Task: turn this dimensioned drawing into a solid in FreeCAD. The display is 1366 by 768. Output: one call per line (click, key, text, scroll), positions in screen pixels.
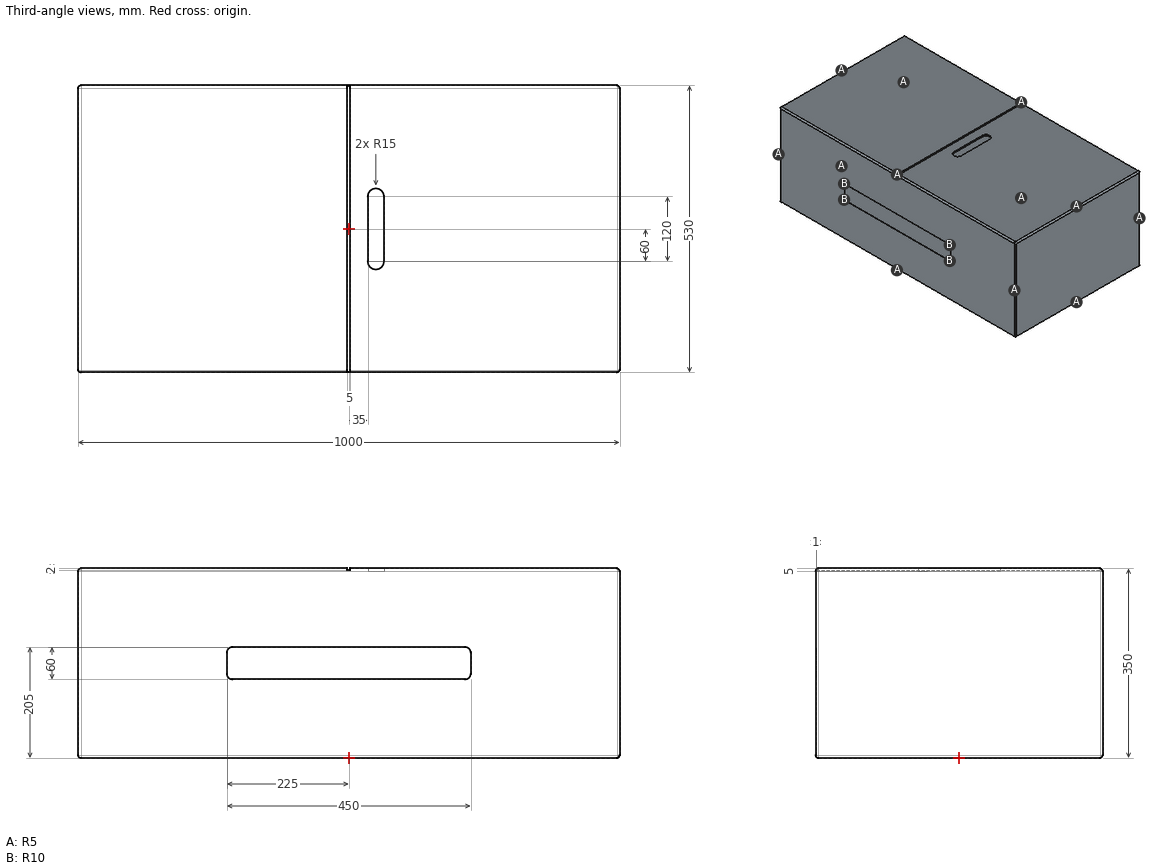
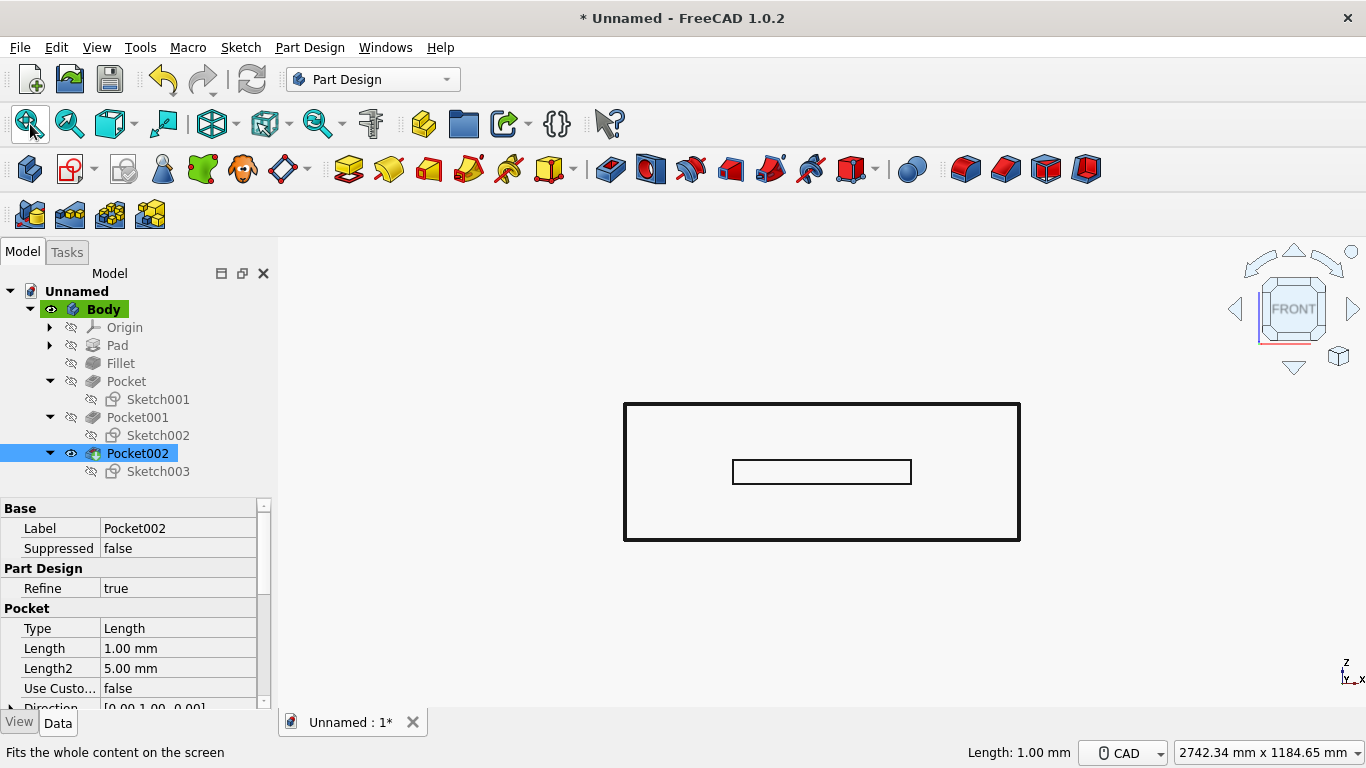
key(3)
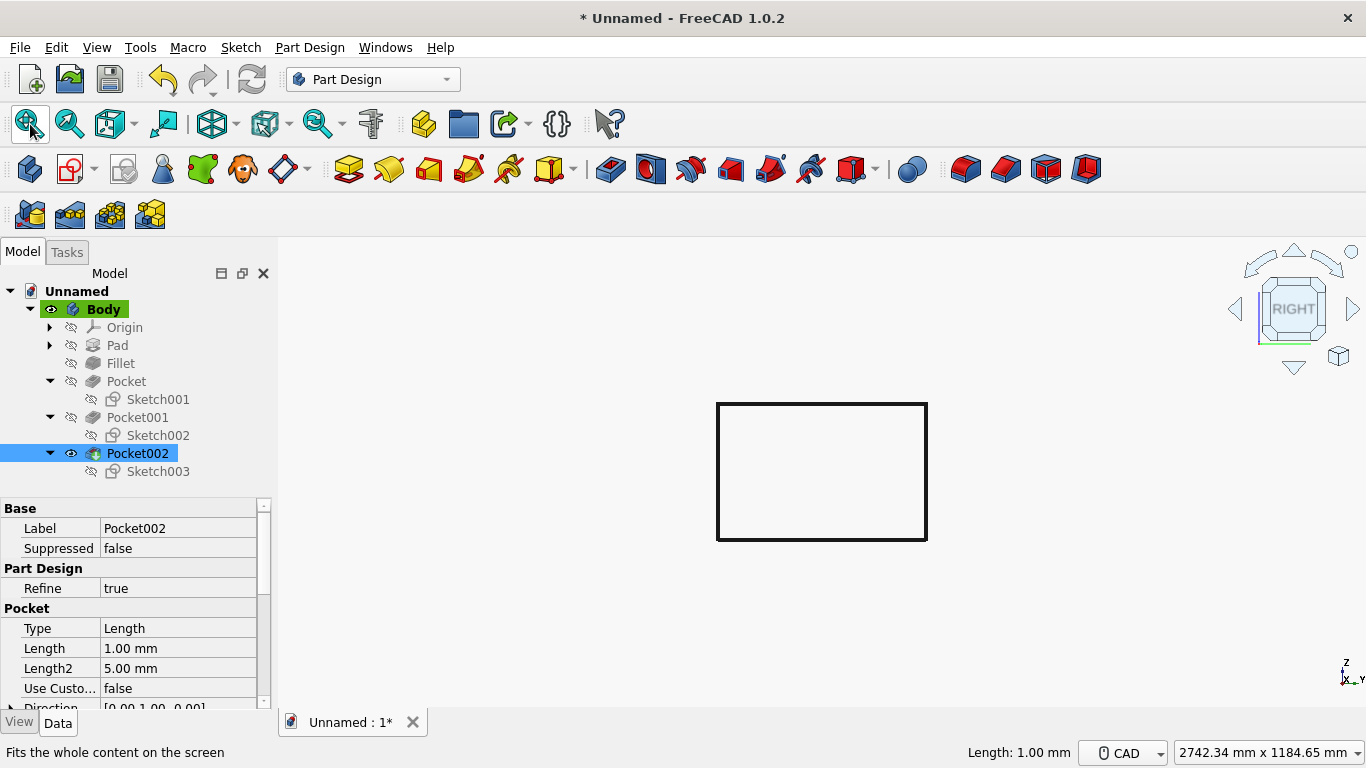
click(30, 124)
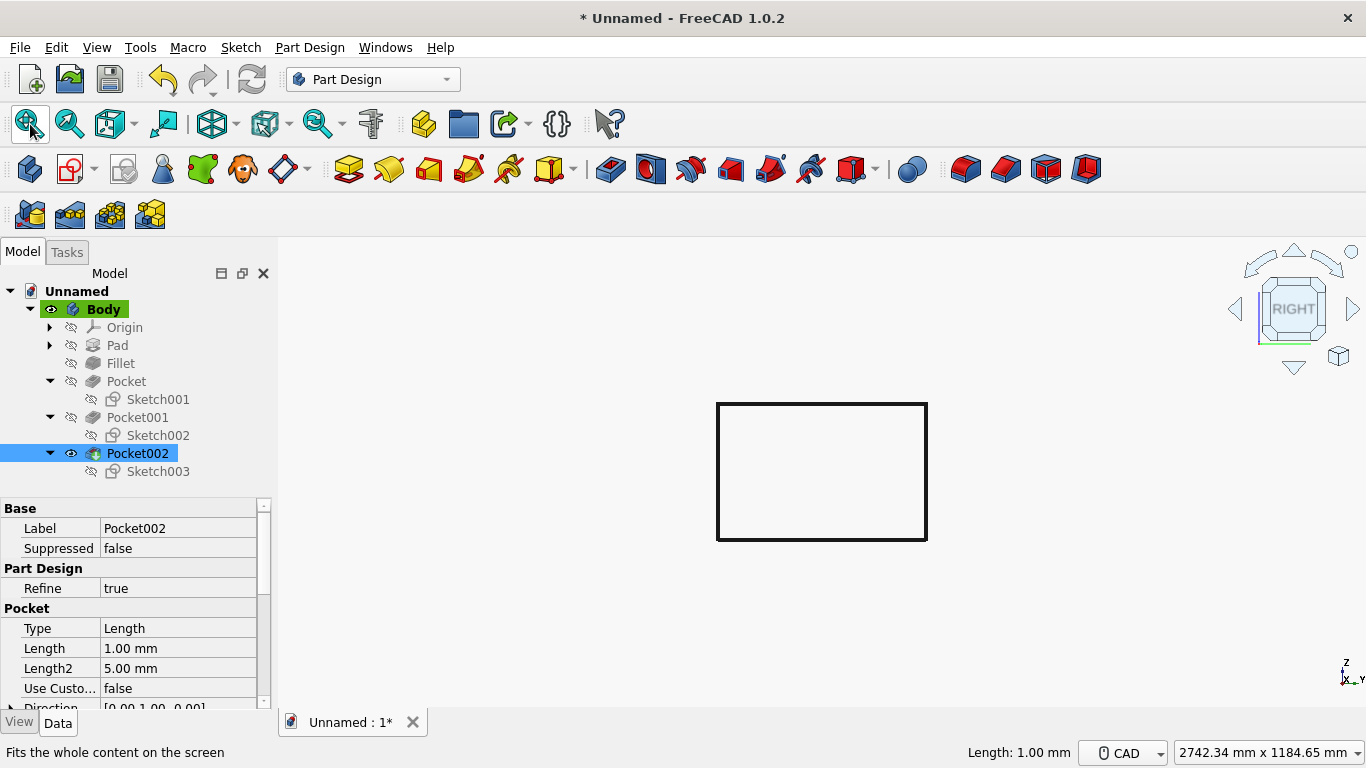
scroll(717, 483, up, 15)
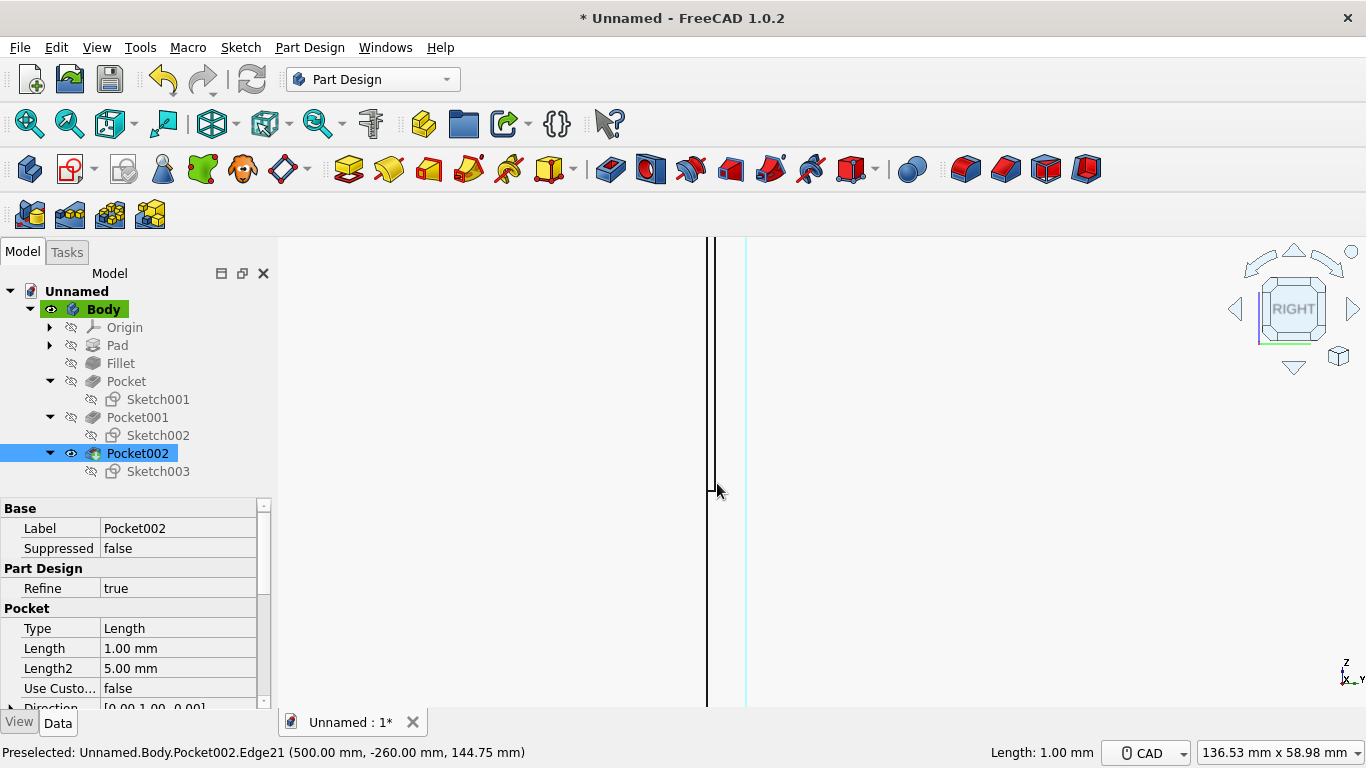
scroll(711, 490, up, 9)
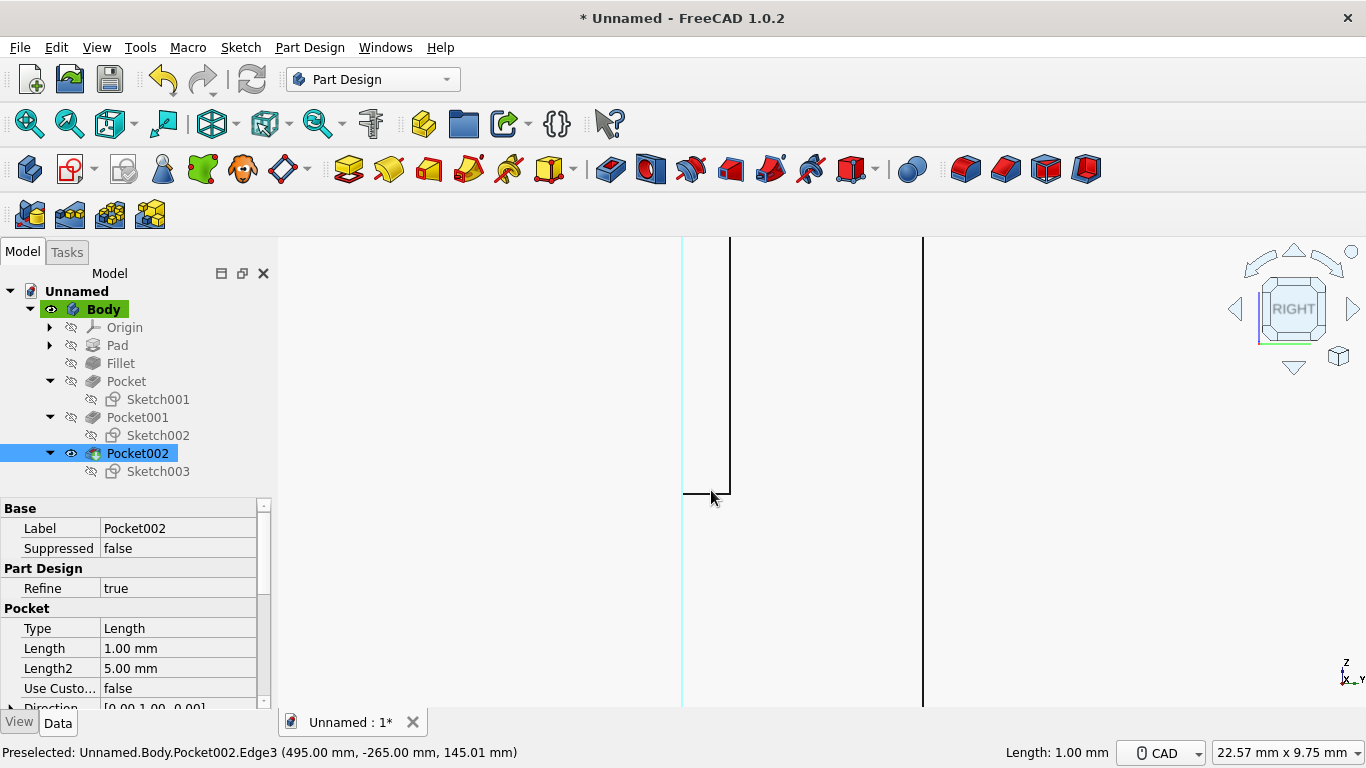
click(706, 493, ctrl)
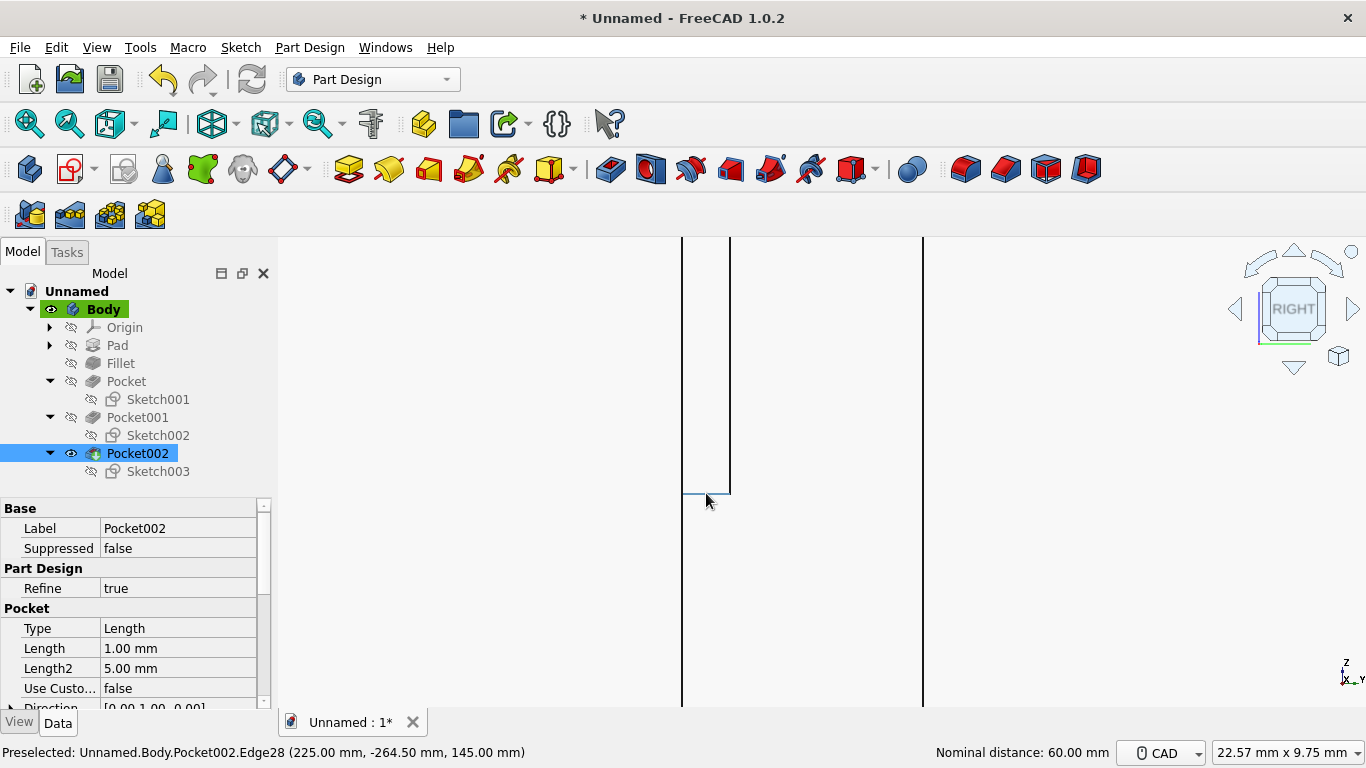
click(30, 124)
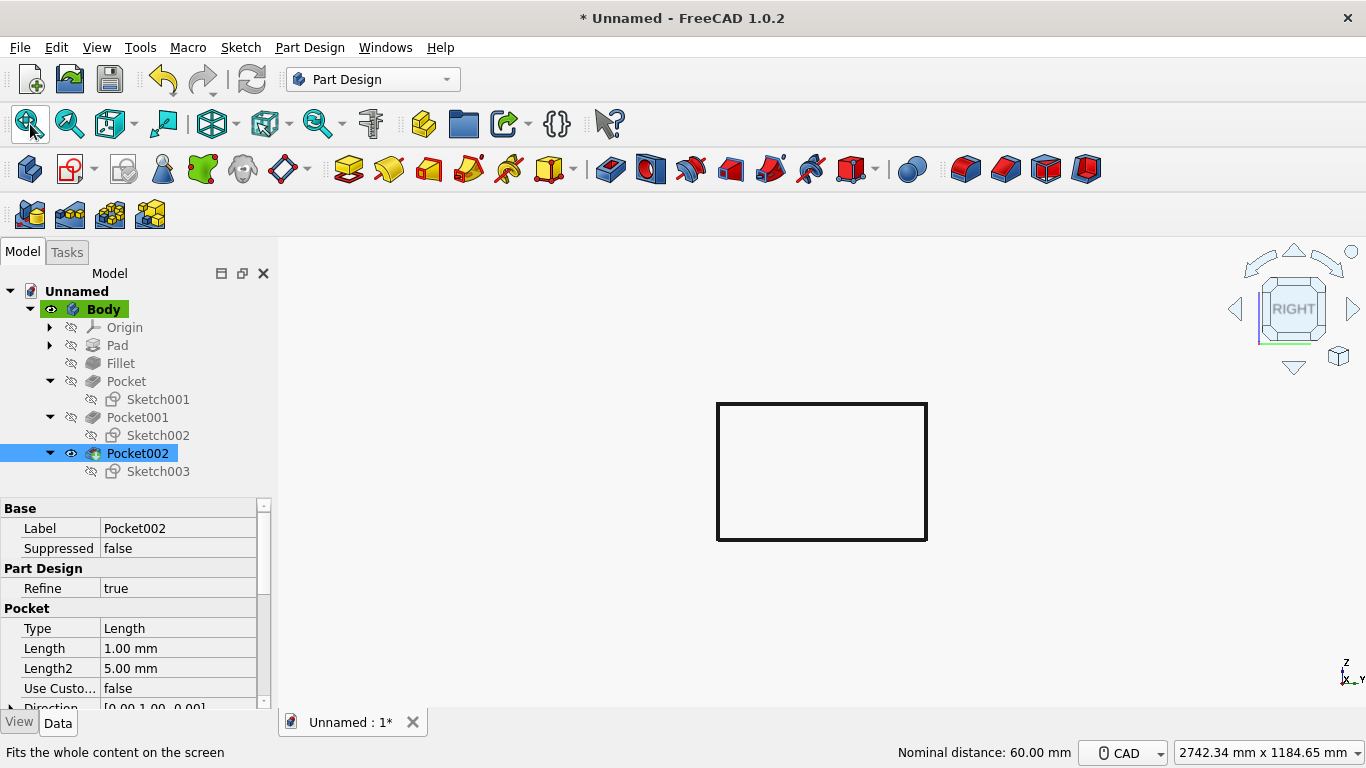
key(5)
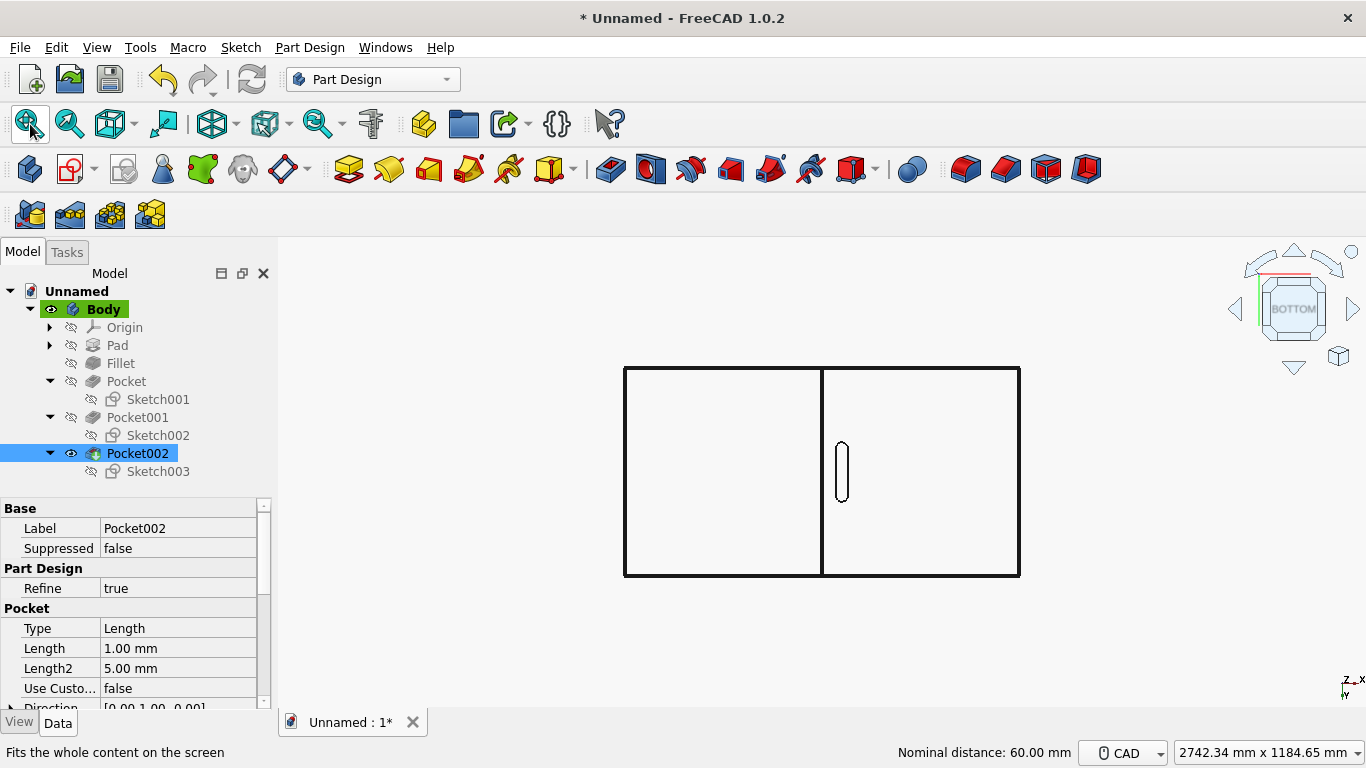
click(30, 124)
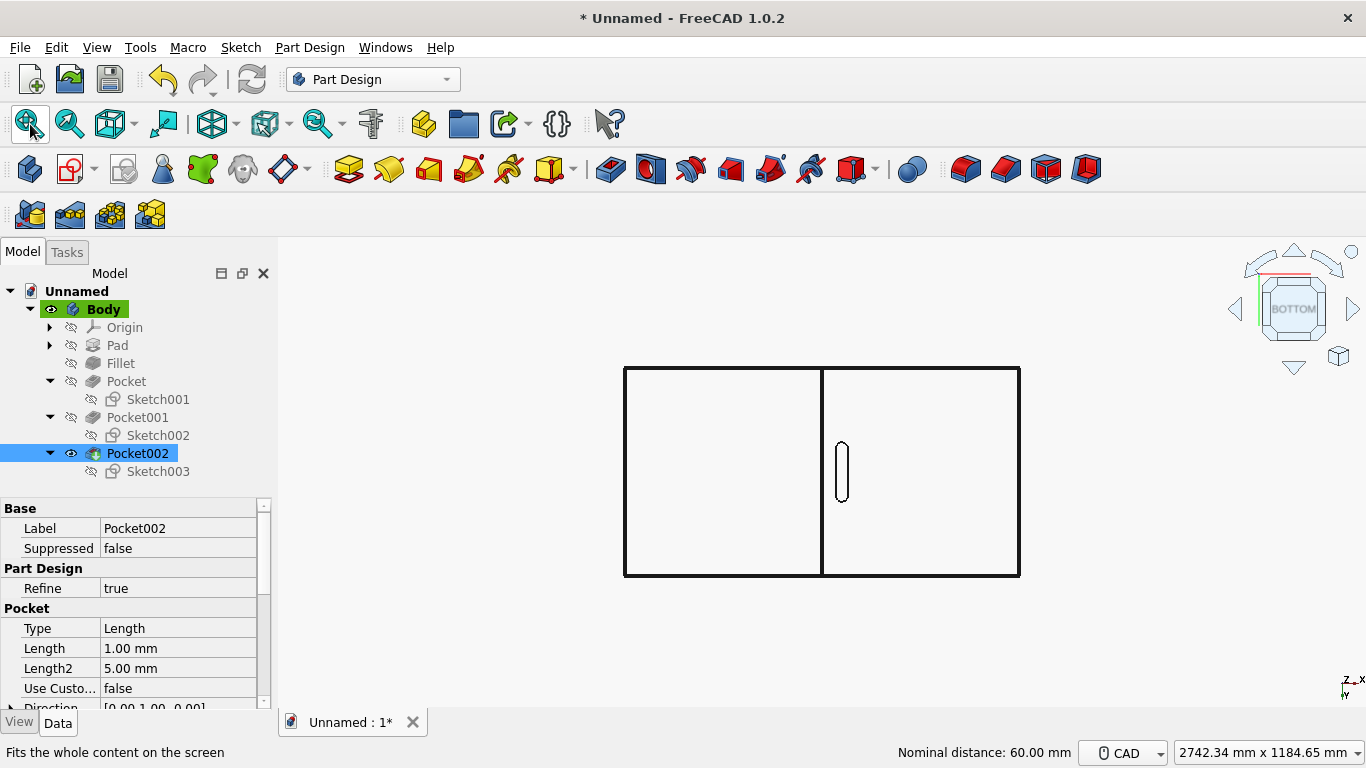
scroll(733, 366, up, 15)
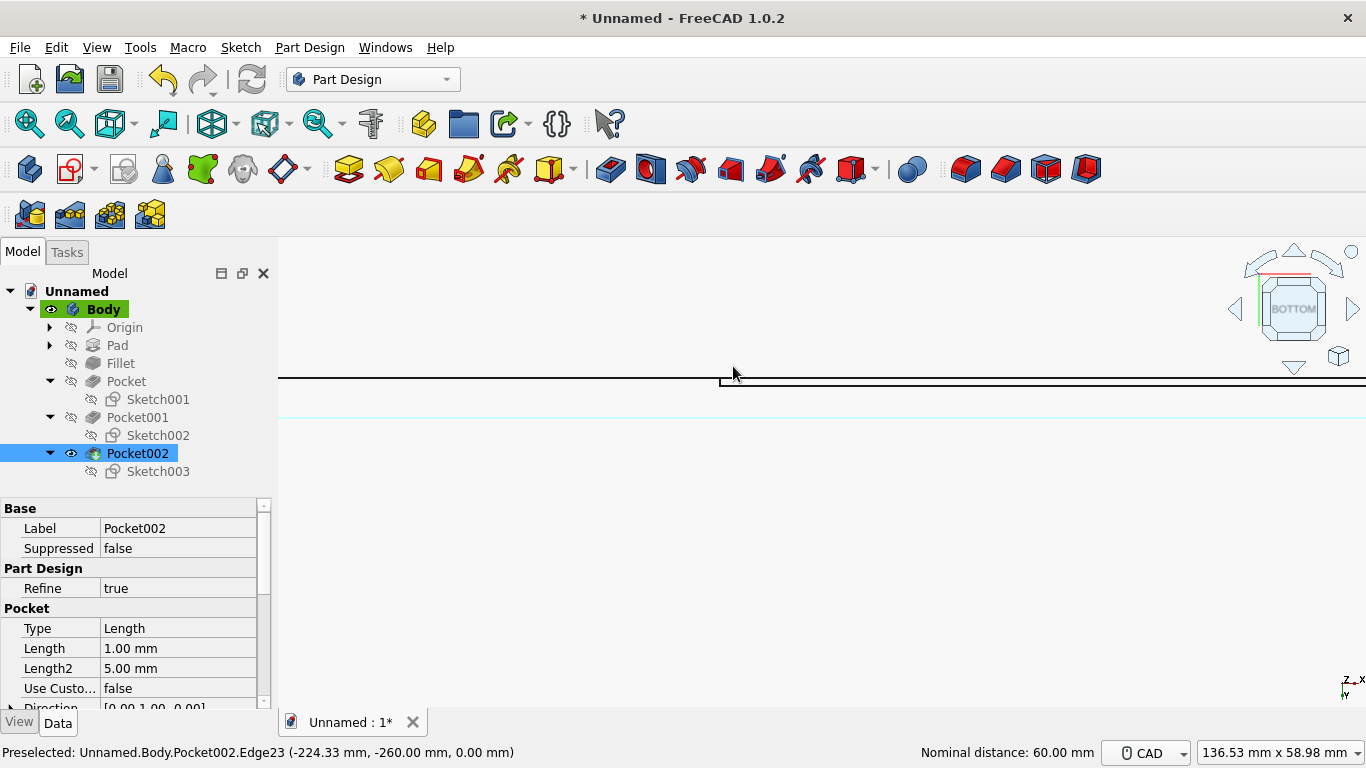
scroll(720, 381, up, 9)